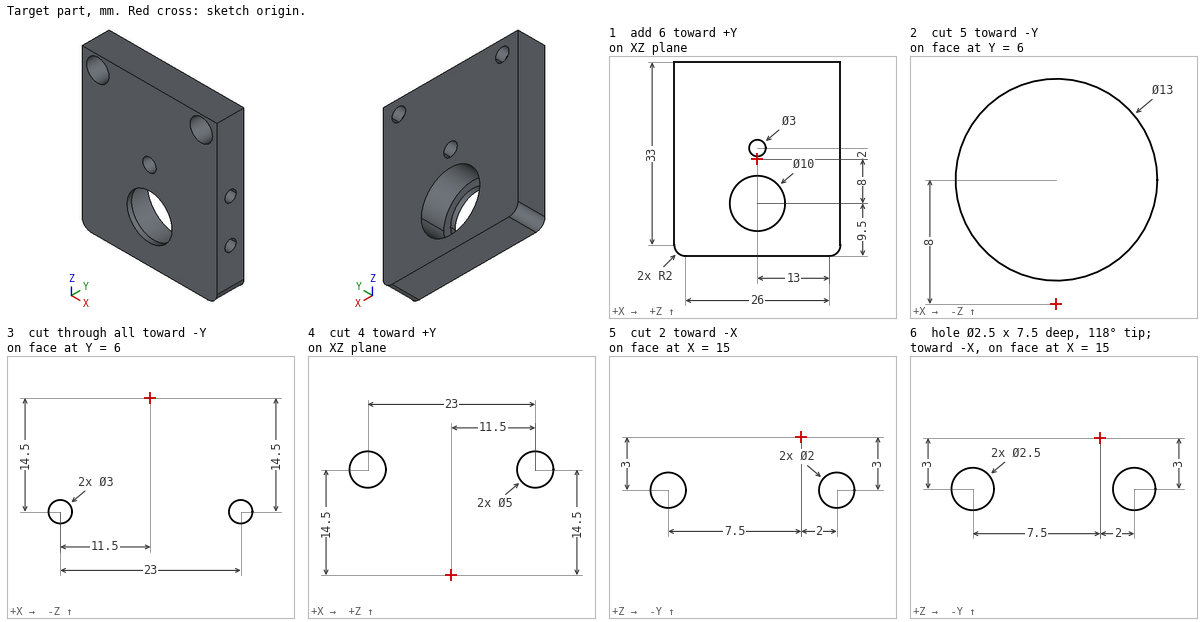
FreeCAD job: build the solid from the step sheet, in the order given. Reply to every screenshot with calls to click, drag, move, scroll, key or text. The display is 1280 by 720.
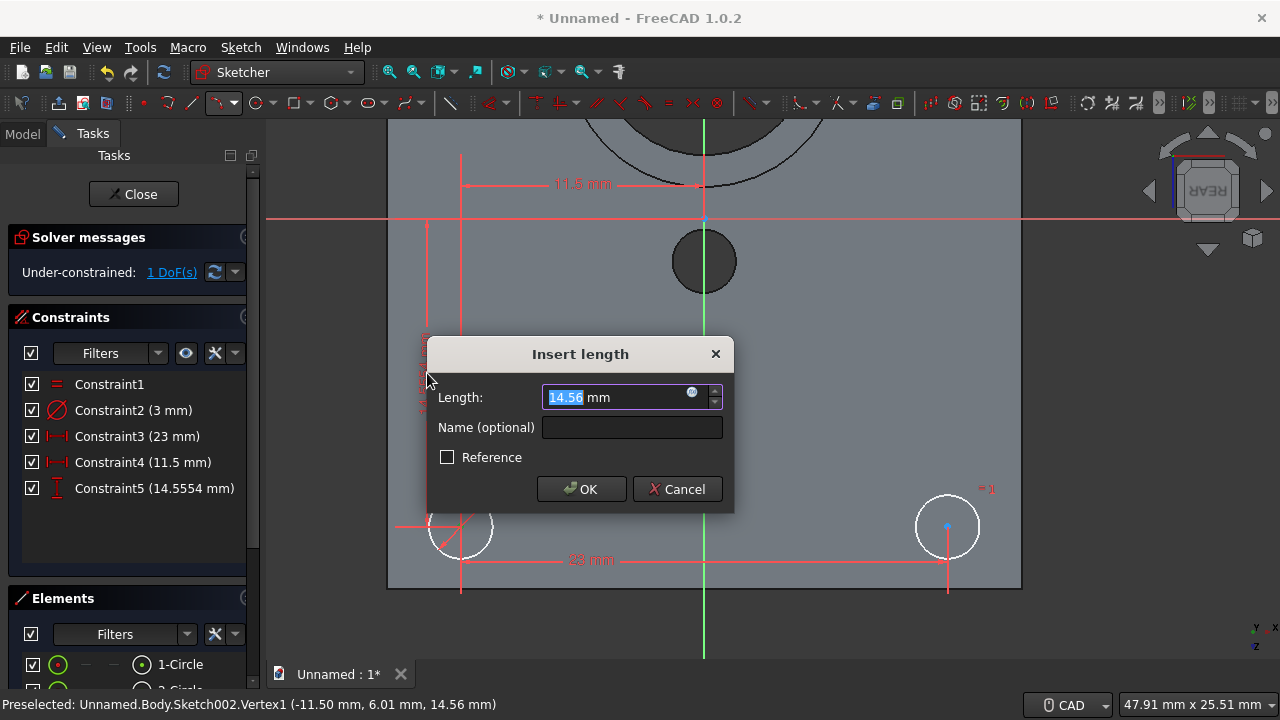
text(14.5)
key(Return)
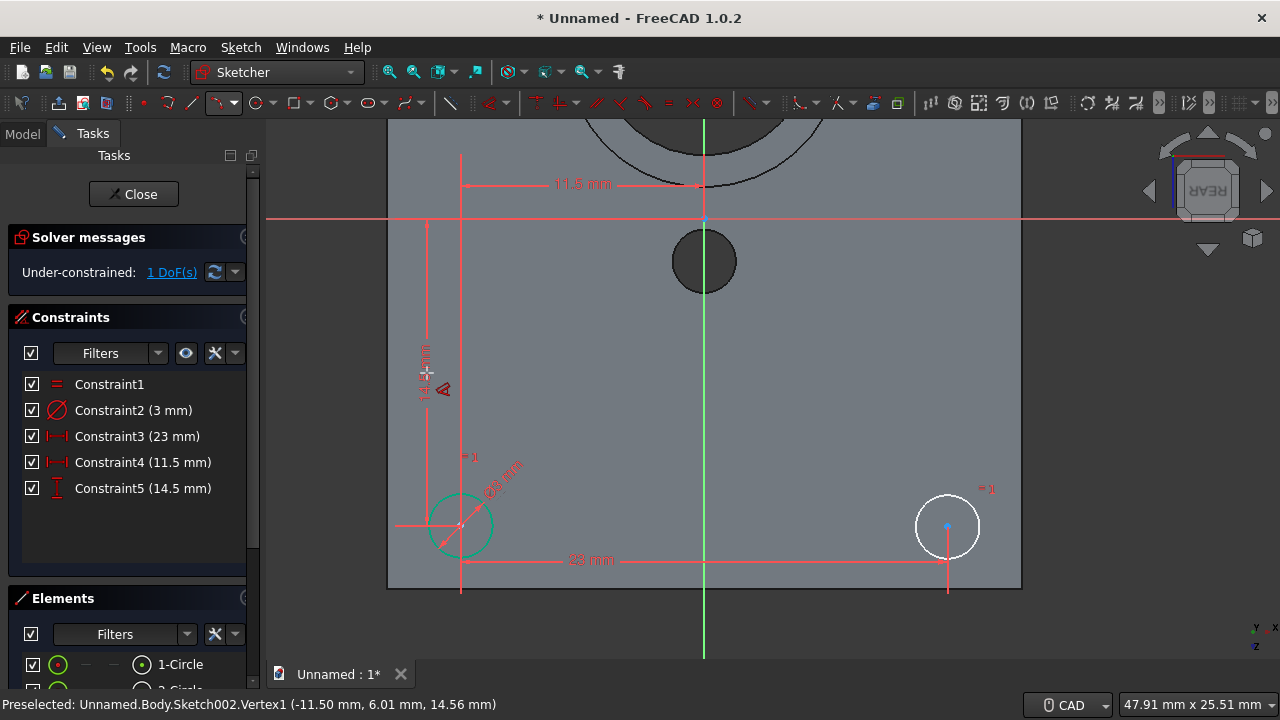
click(948, 527)
click(982, 373)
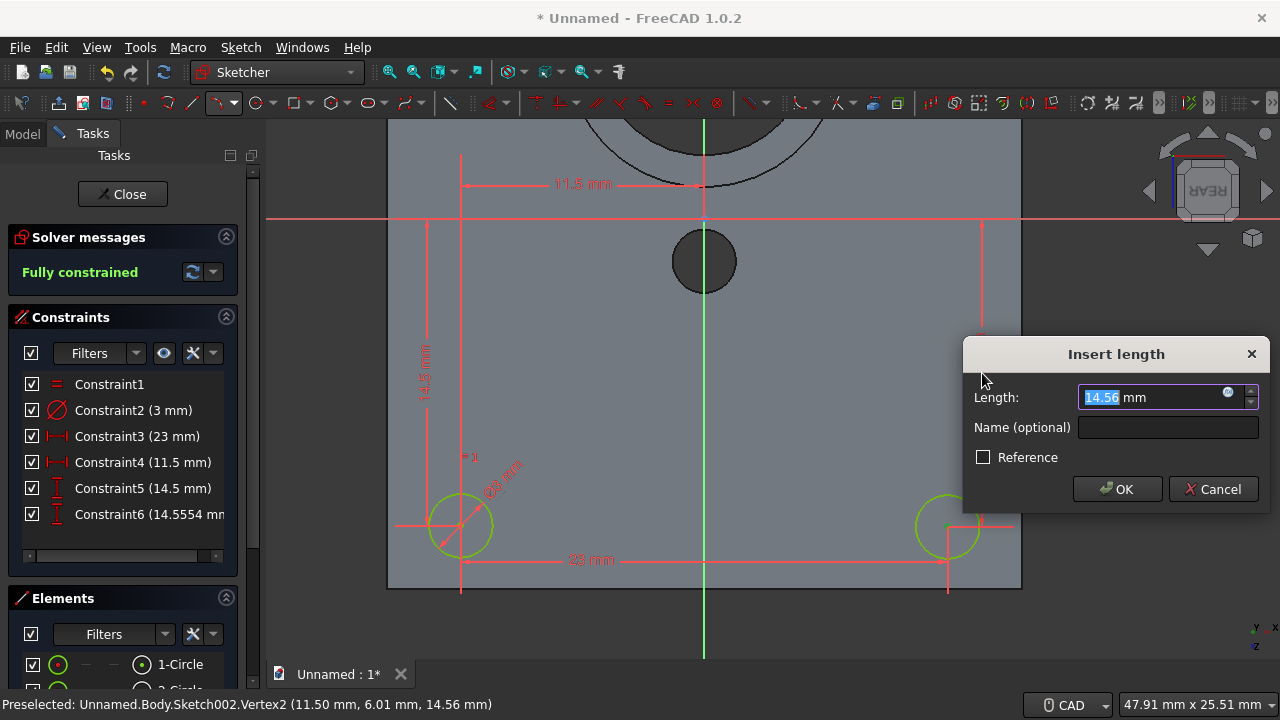
text(14.5)
key(Return)
key(Escape)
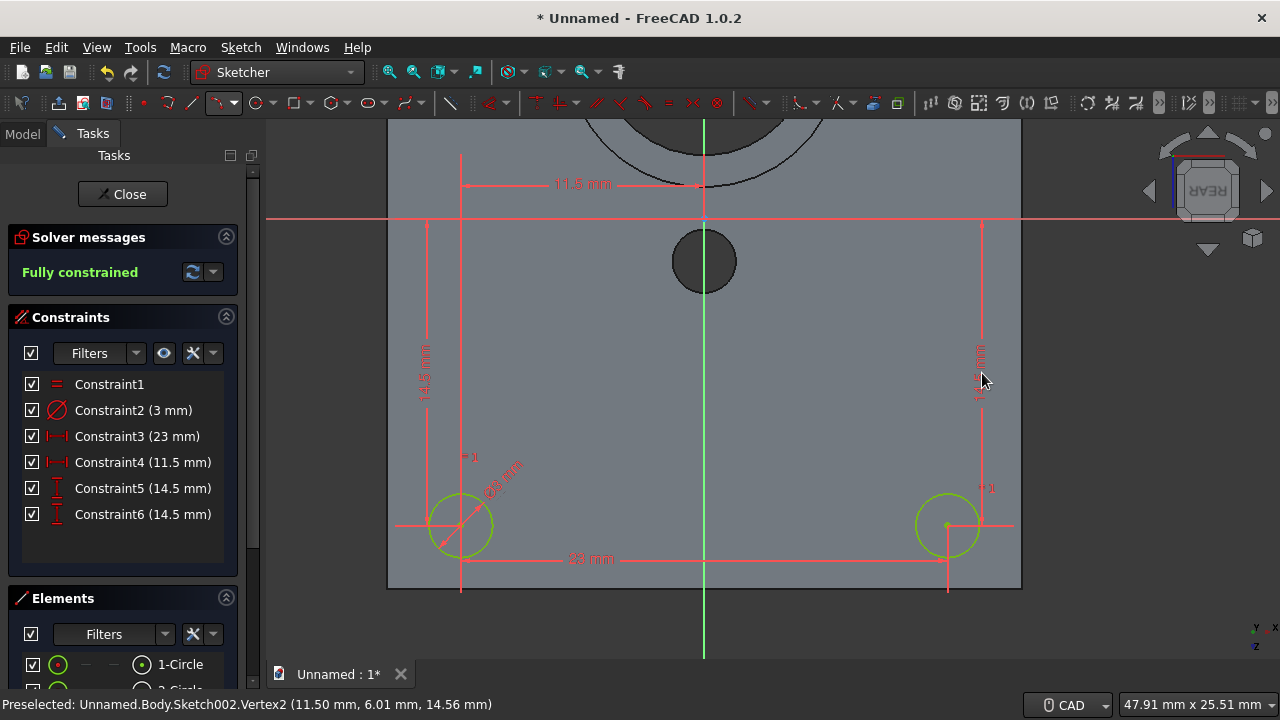
click(123, 194)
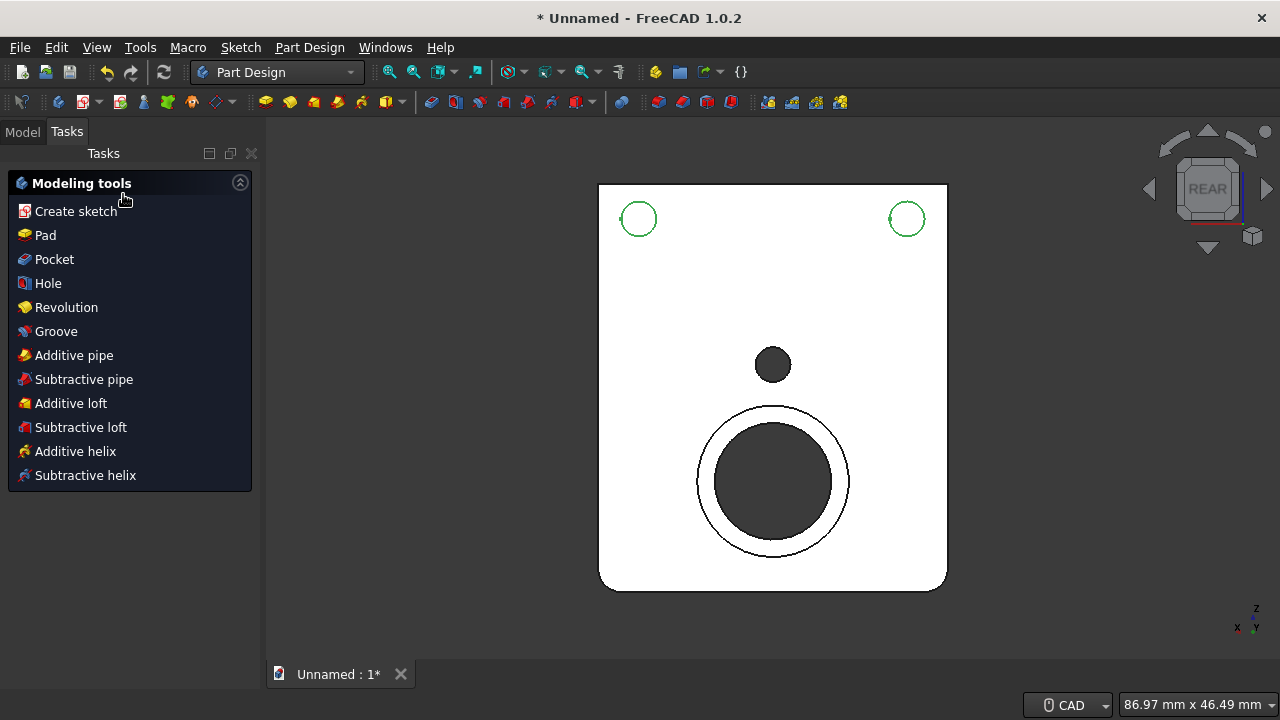
click(432, 102)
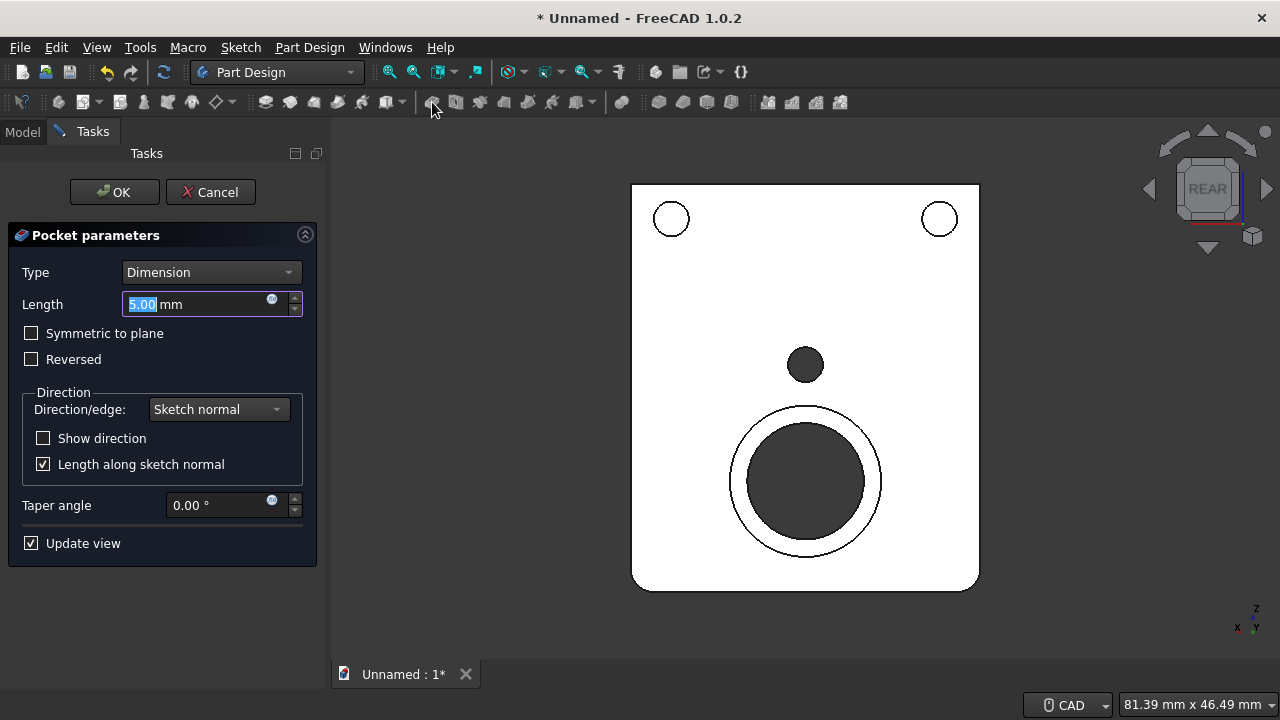
click(212, 272)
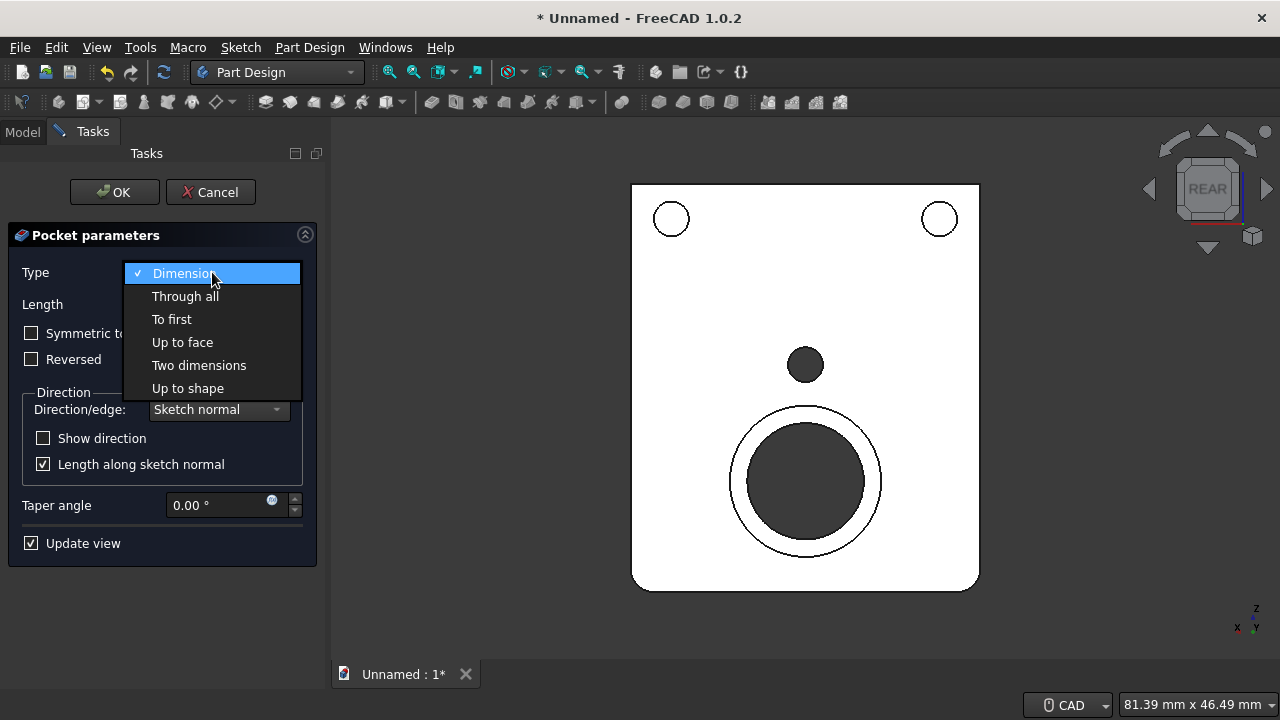
click(212, 296)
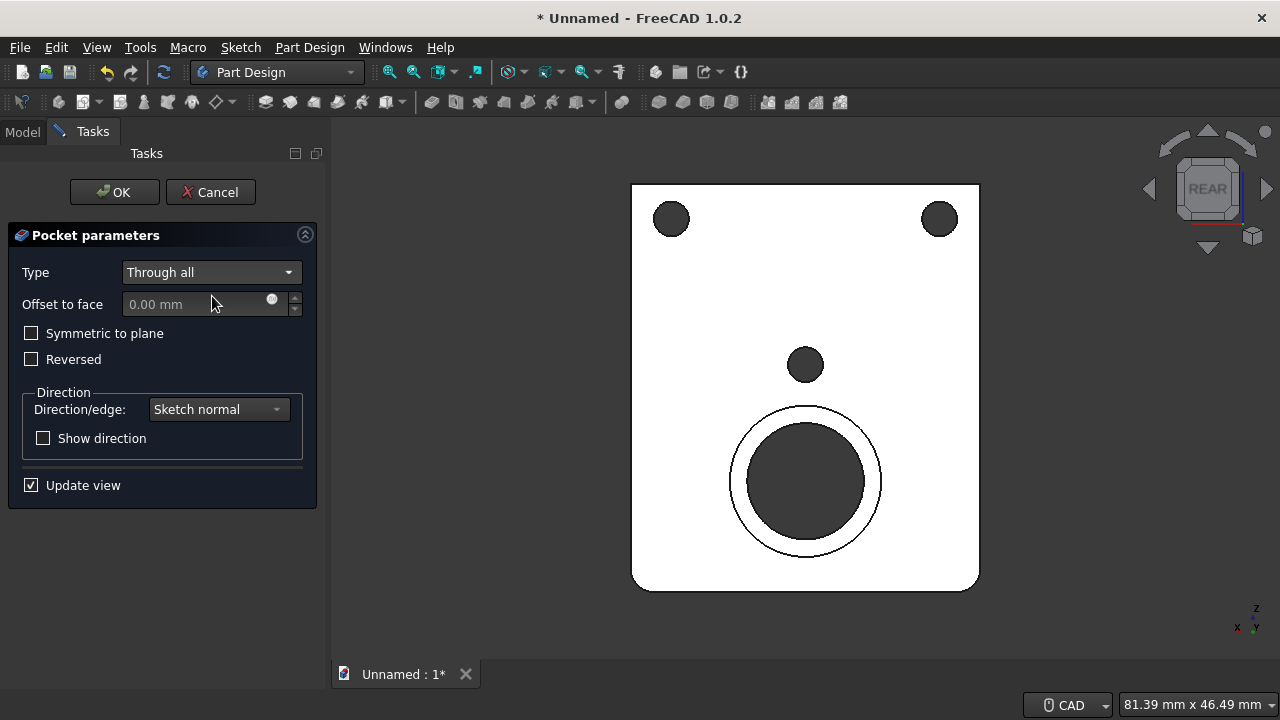
click(115, 192)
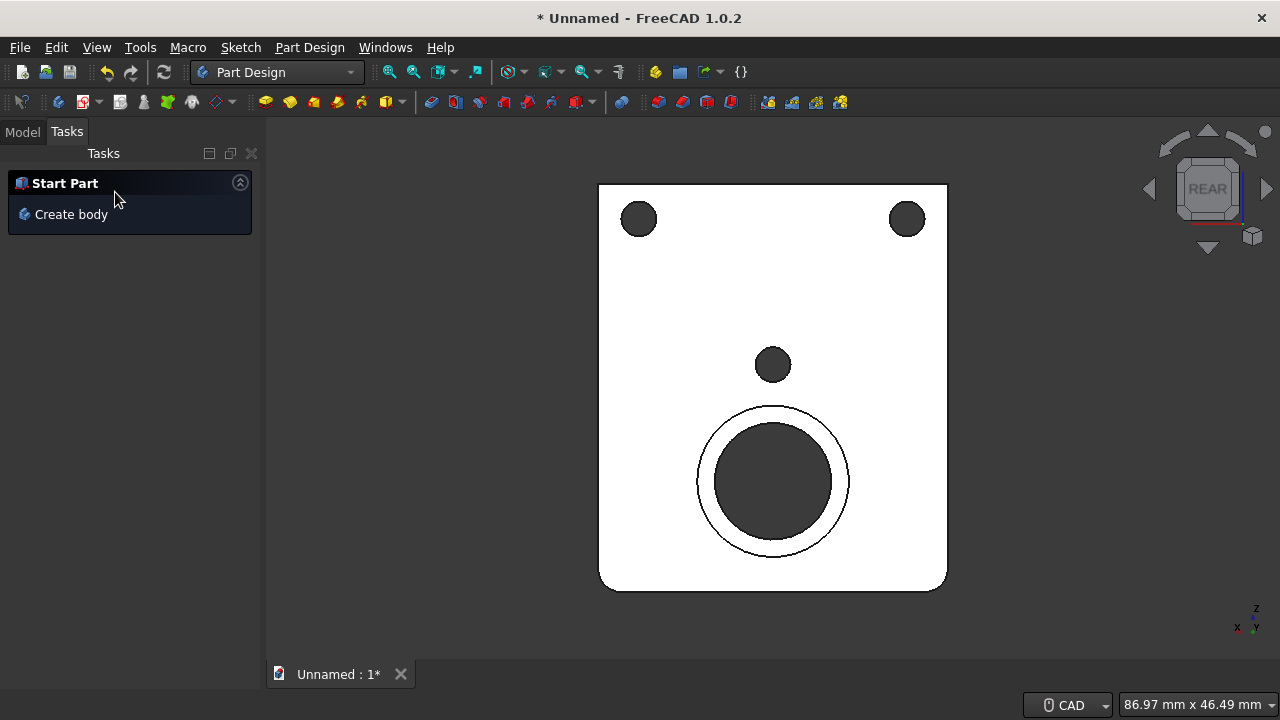
click(84, 102)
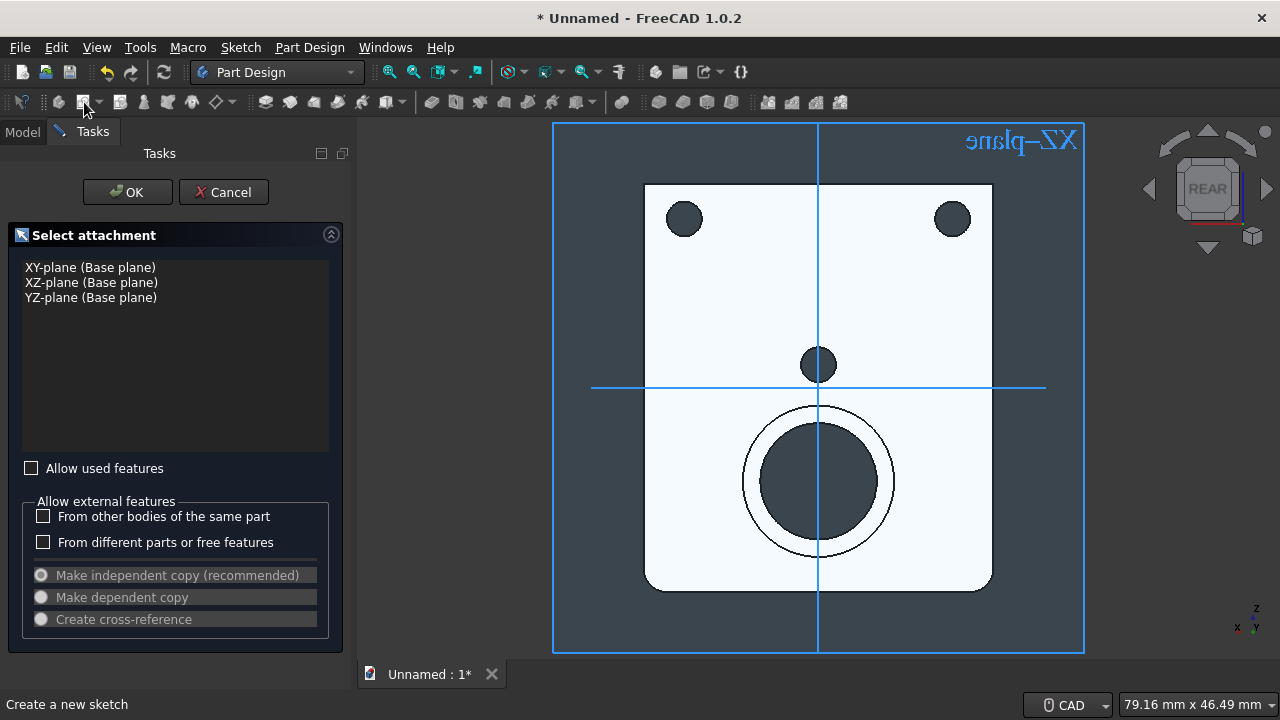
click(82, 282)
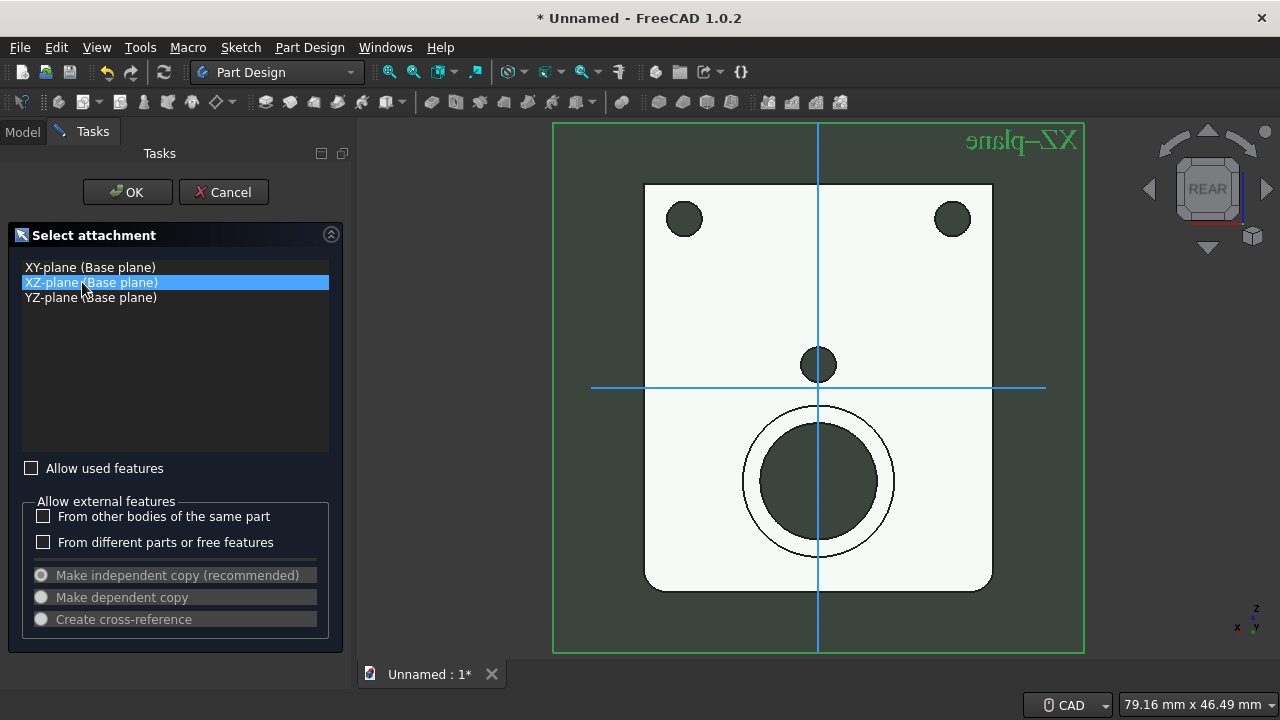
click(128, 192)